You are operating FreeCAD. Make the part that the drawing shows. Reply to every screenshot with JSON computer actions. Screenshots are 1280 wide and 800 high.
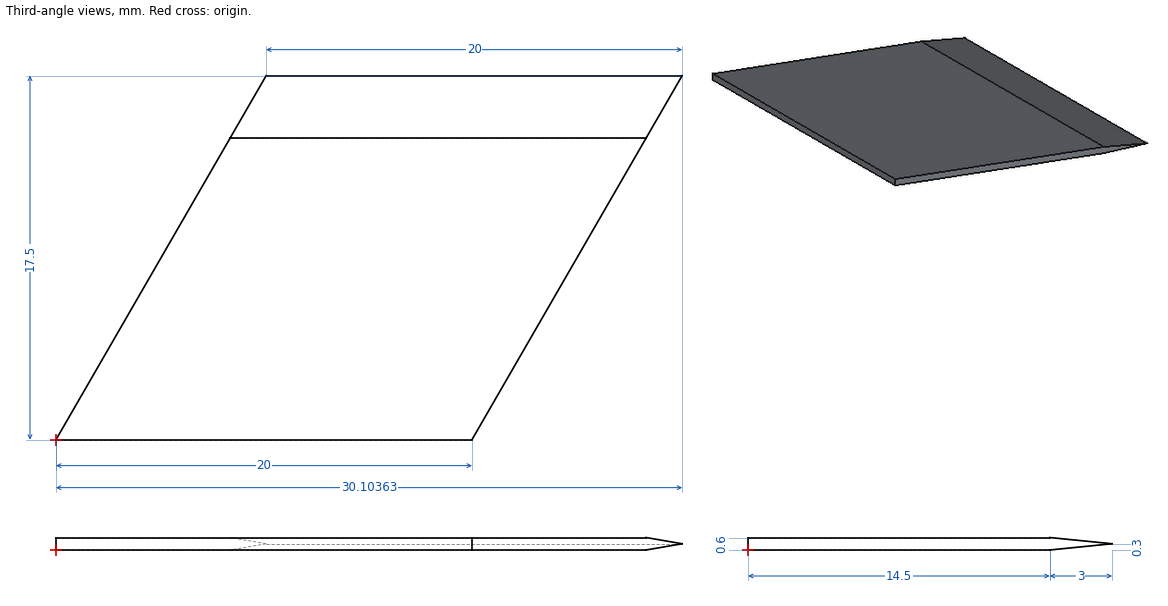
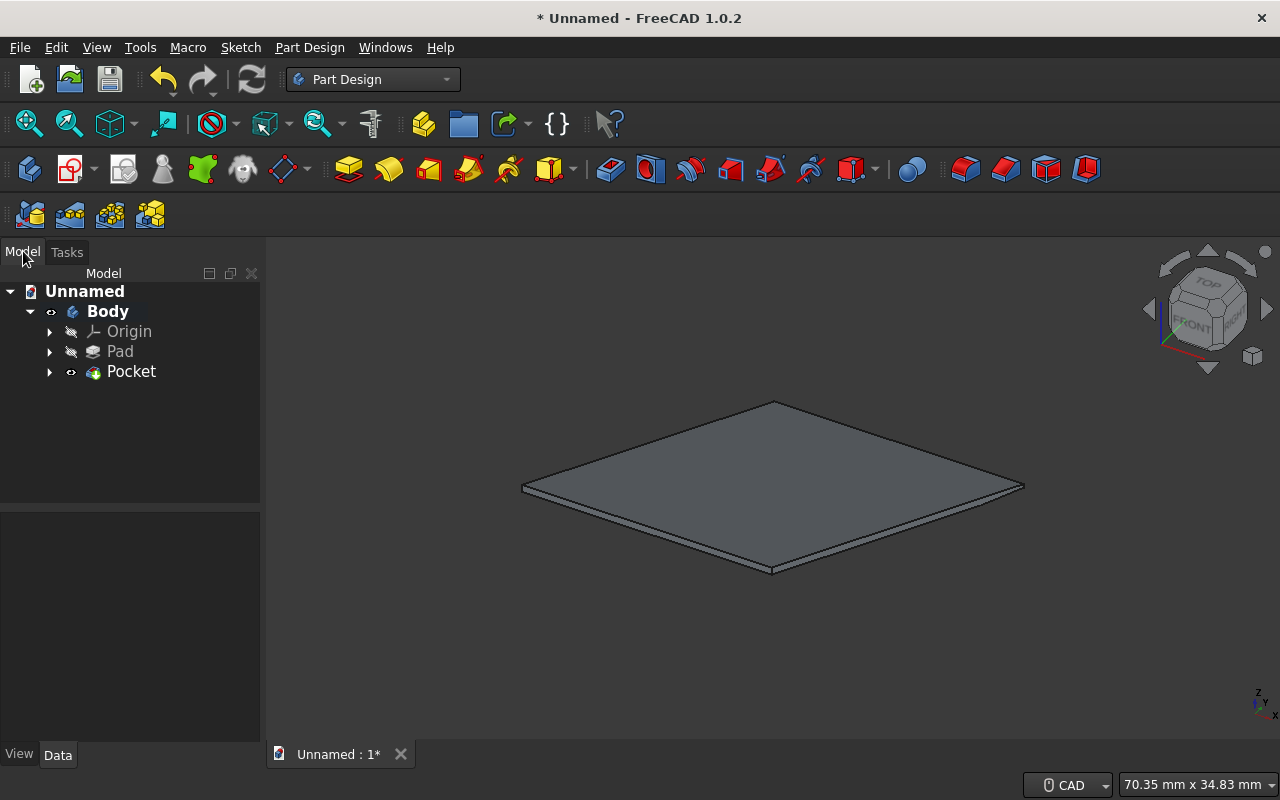
{"action": "left_click", "coordinate": [50, 332]}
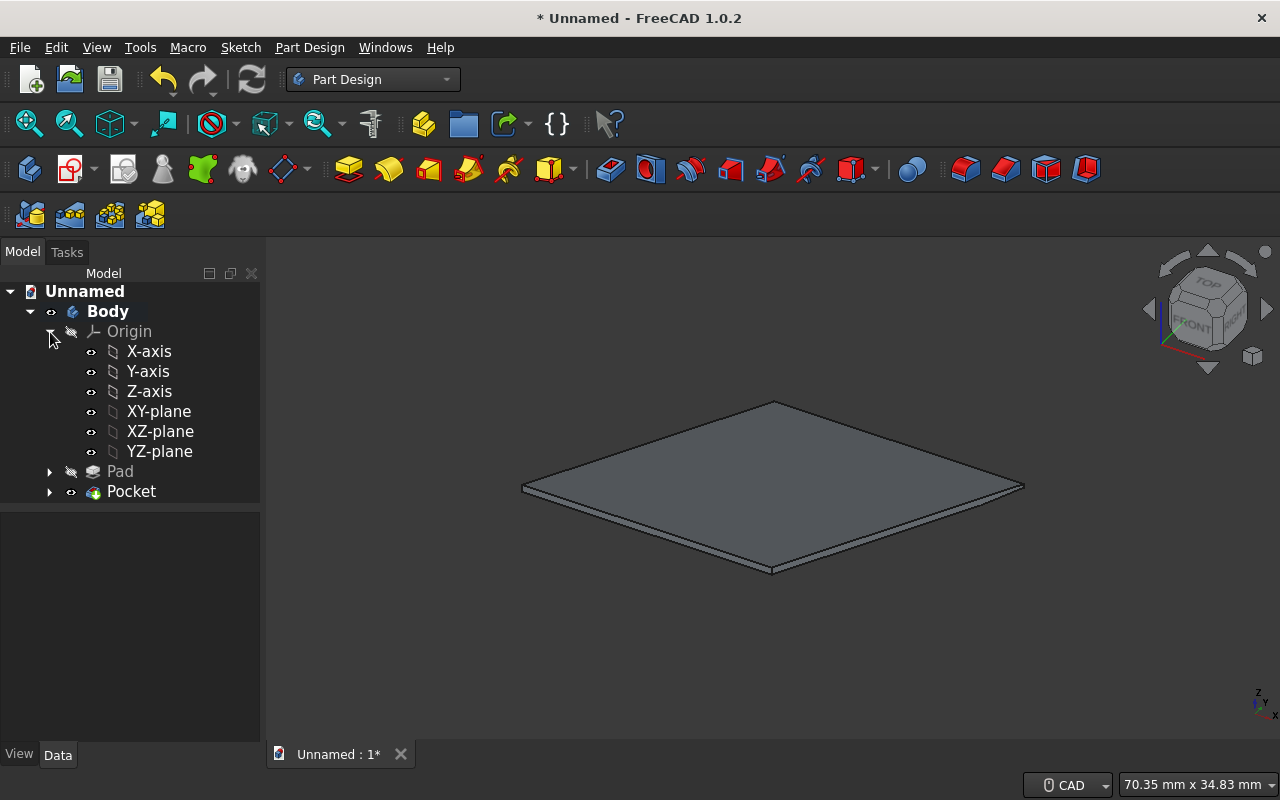
{"action": "left_click", "coordinate": [136, 412]}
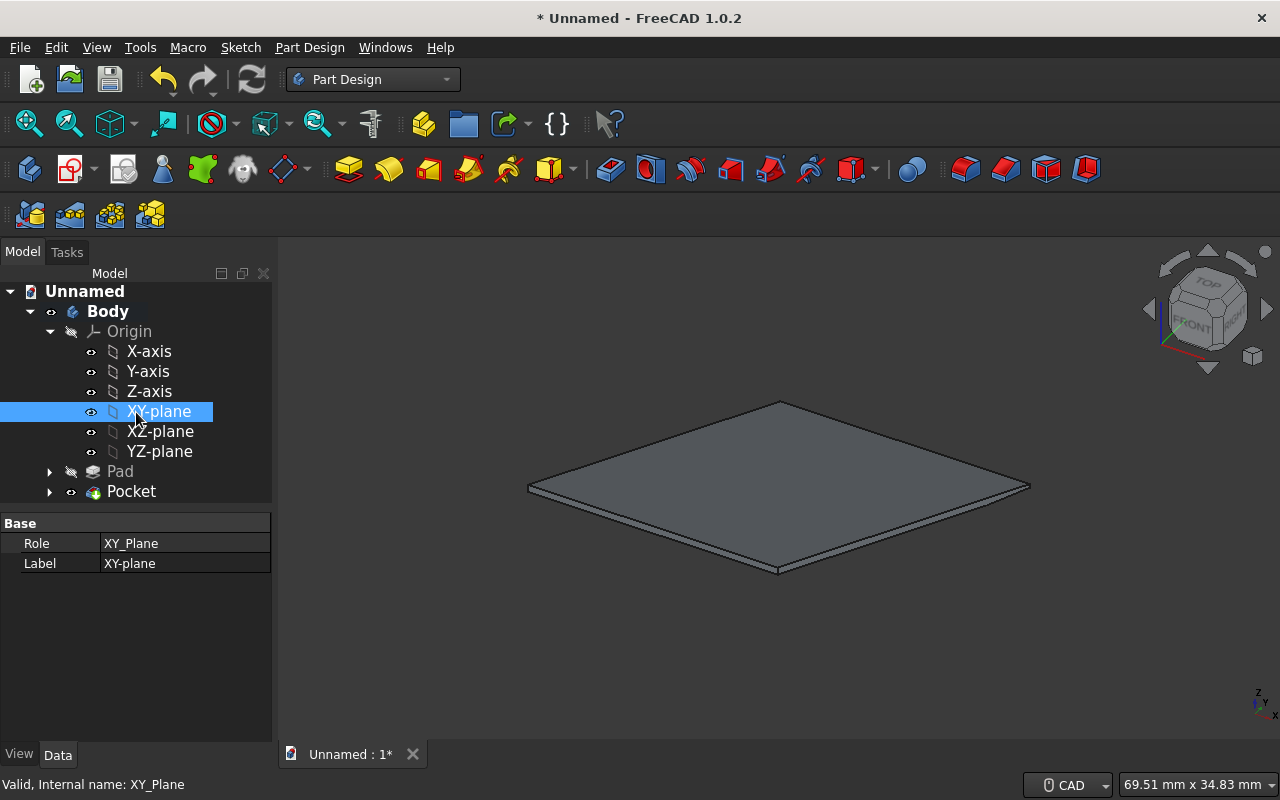
{"action": "left_click", "coordinate": [284, 170]}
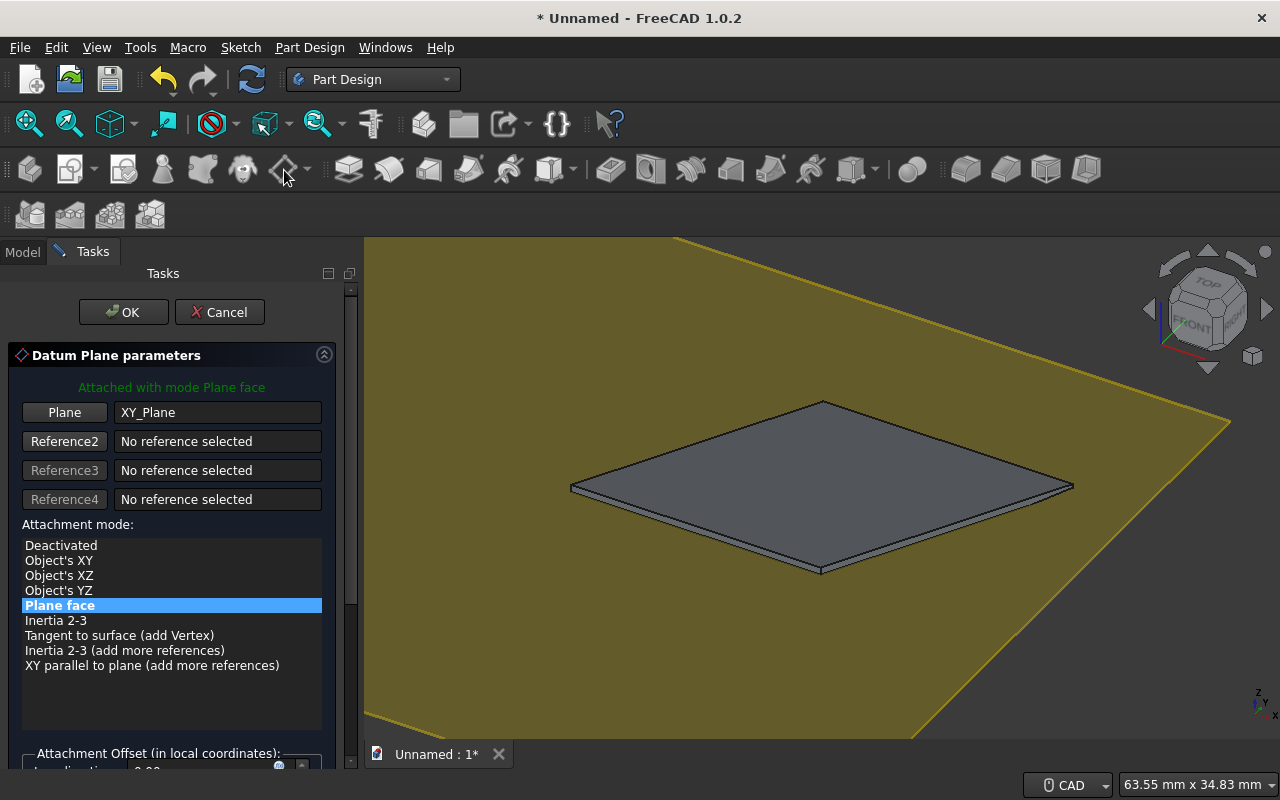
{"action": "scroll", "coordinate": [351, 526], "scroll_direction": "down", "scroll_amount": 3}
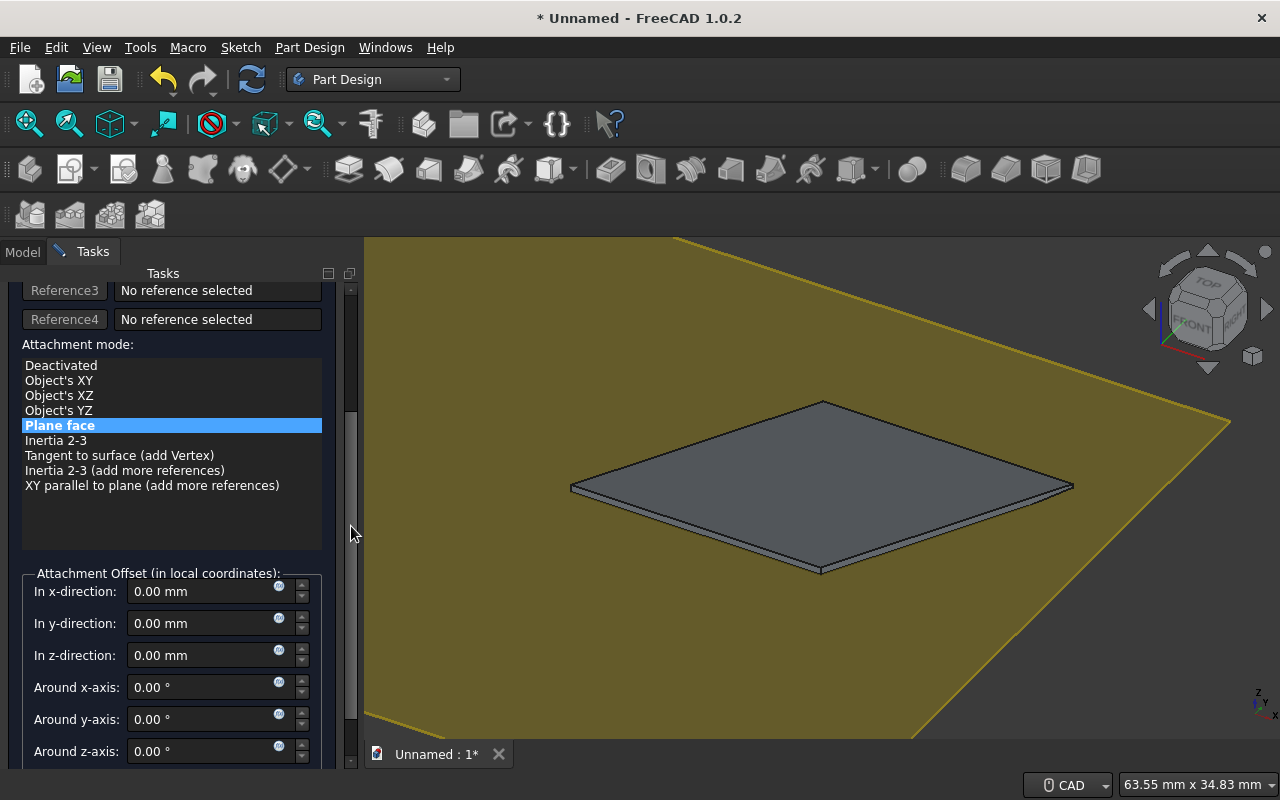
{"action": "triple_click", "coordinate": [210, 655]}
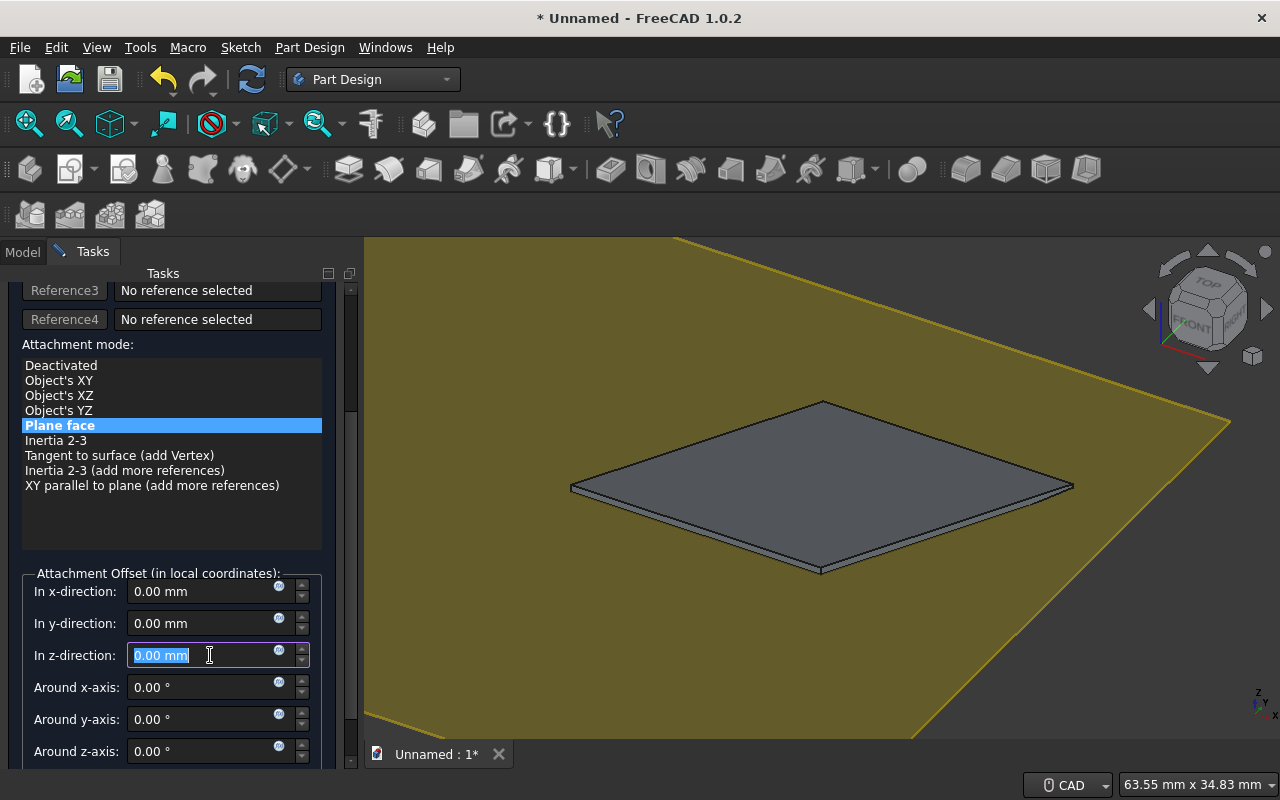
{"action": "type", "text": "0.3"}
{"action": "key", "text": "Tab"}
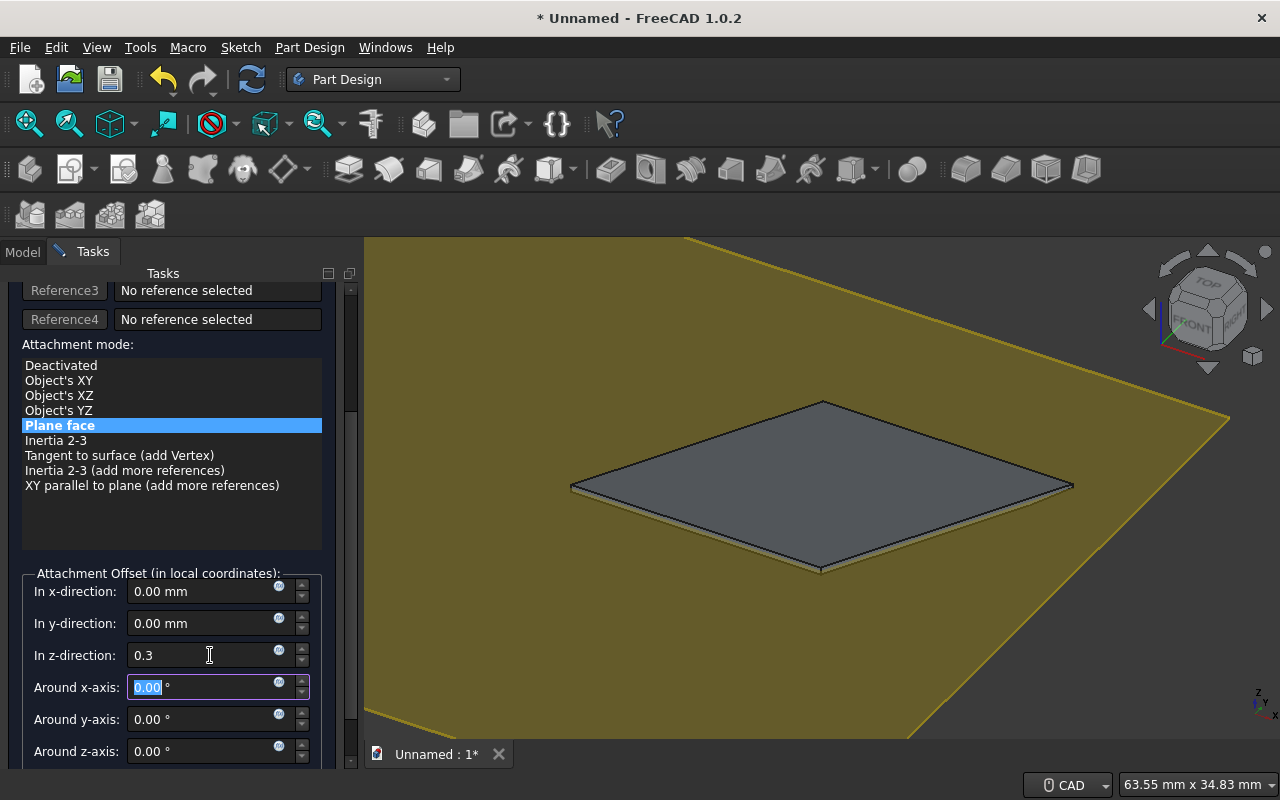
{"action": "scroll", "coordinate": [351, 526], "scroll_direction": "up", "scroll_amount": 4}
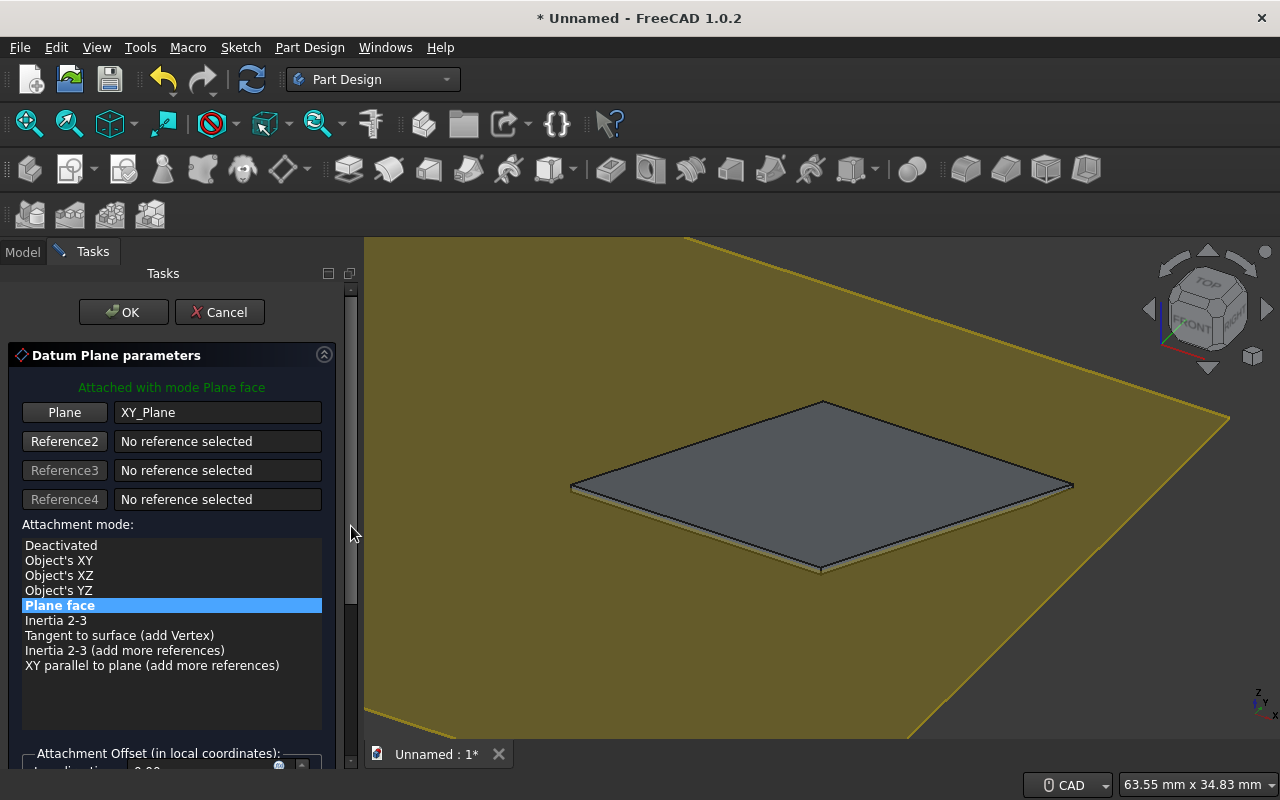
{"action": "left_click", "coordinate": [124, 312]}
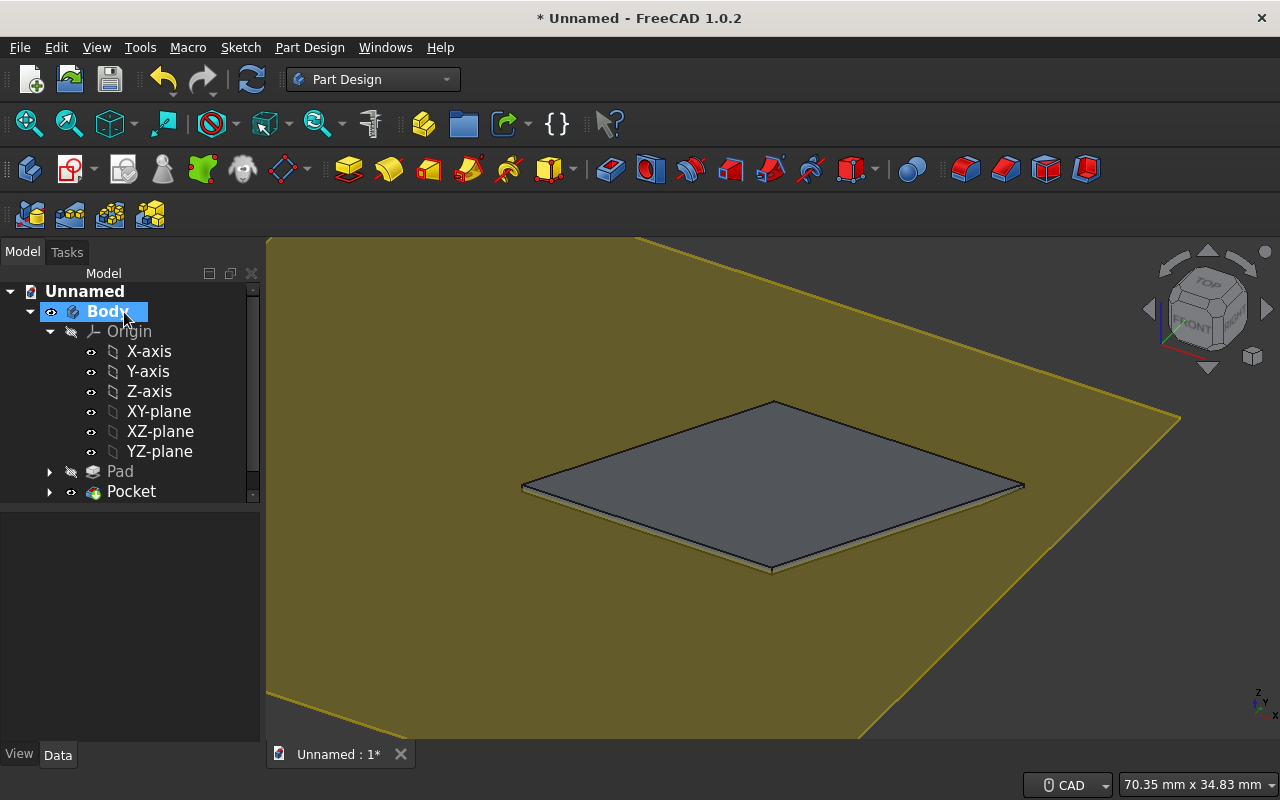
{"action": "left_click", "coordinate": [116, 492]}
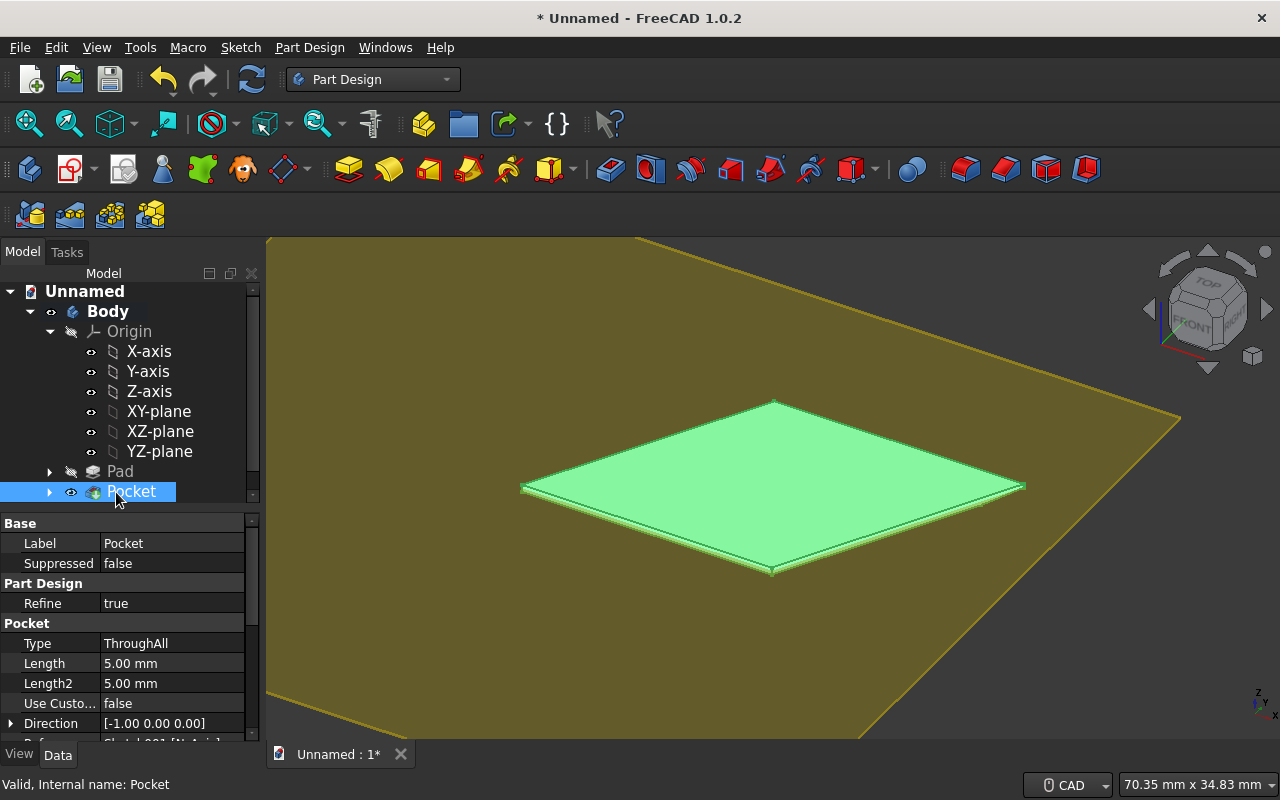
{"action": "left_click", "coordinate": [30, 214]}